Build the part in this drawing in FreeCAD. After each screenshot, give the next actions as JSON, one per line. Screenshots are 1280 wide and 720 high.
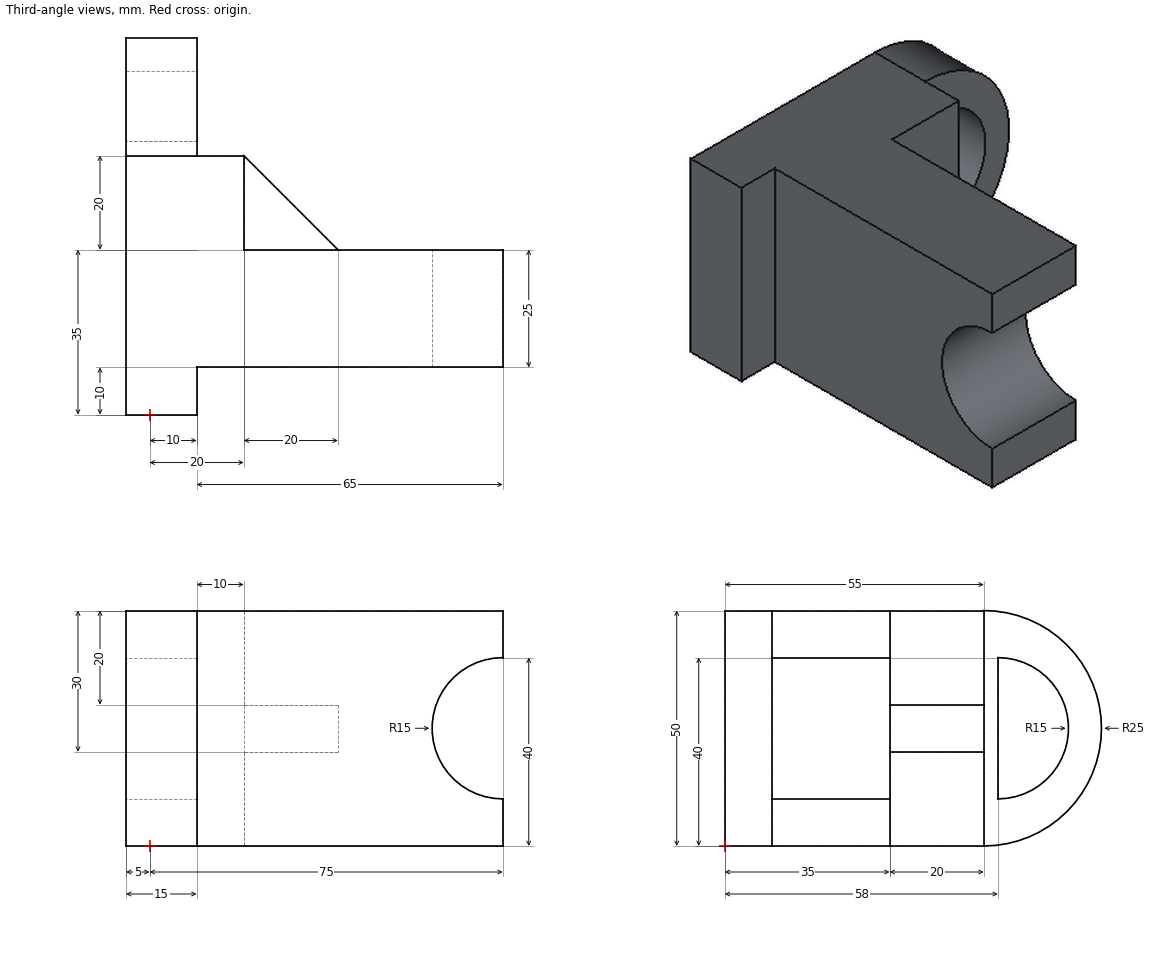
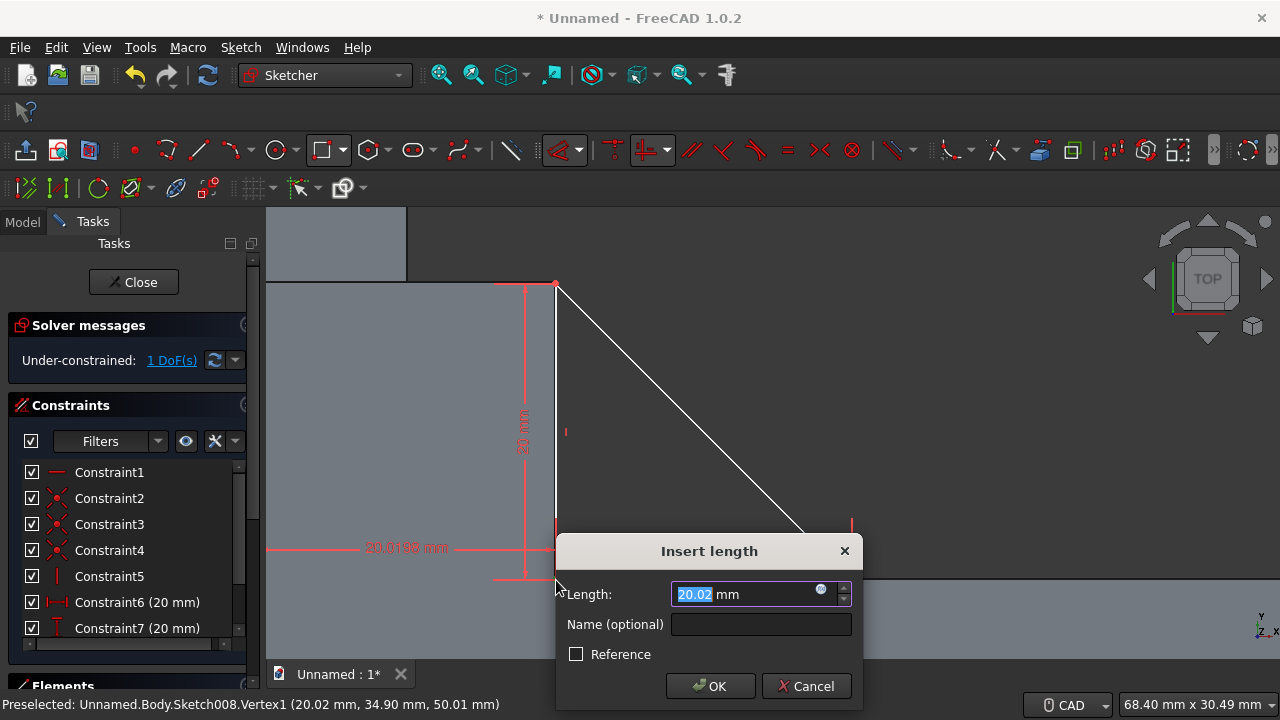
{"action": "type", "text": "20"}
{"action": "key", "text": "Return"}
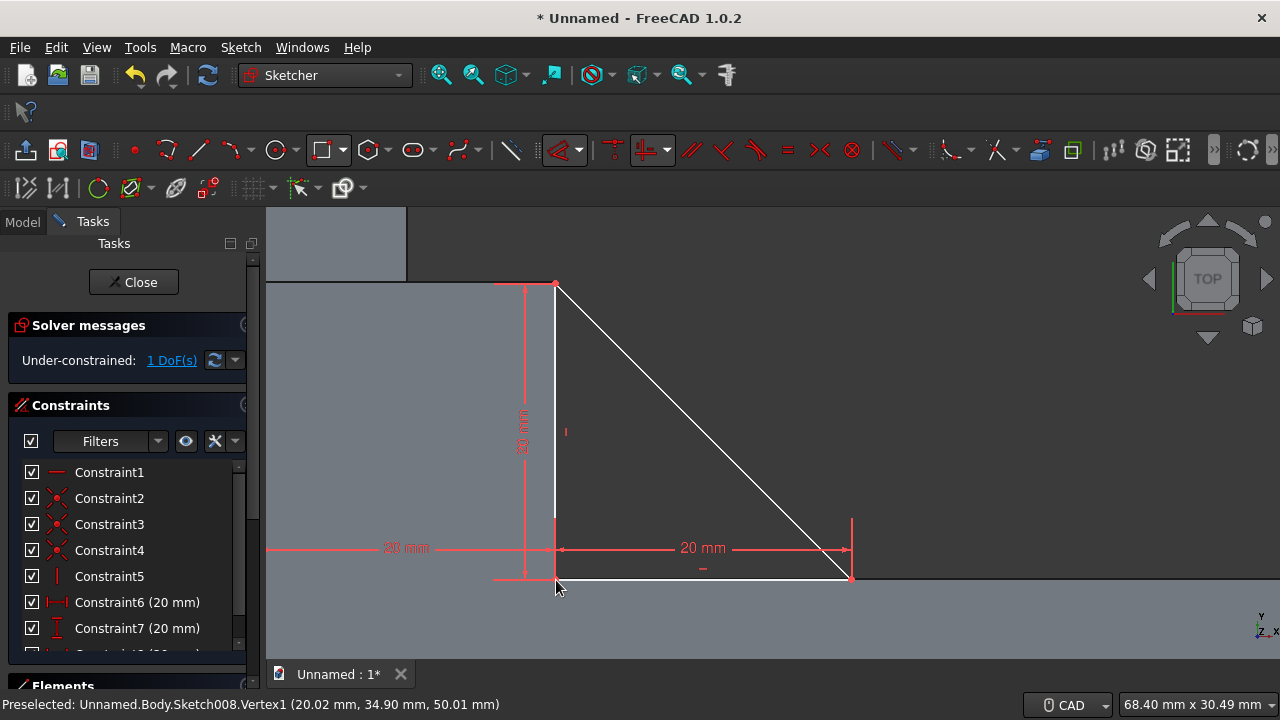
{"action": "left_click", "coordinate": [555, 580]}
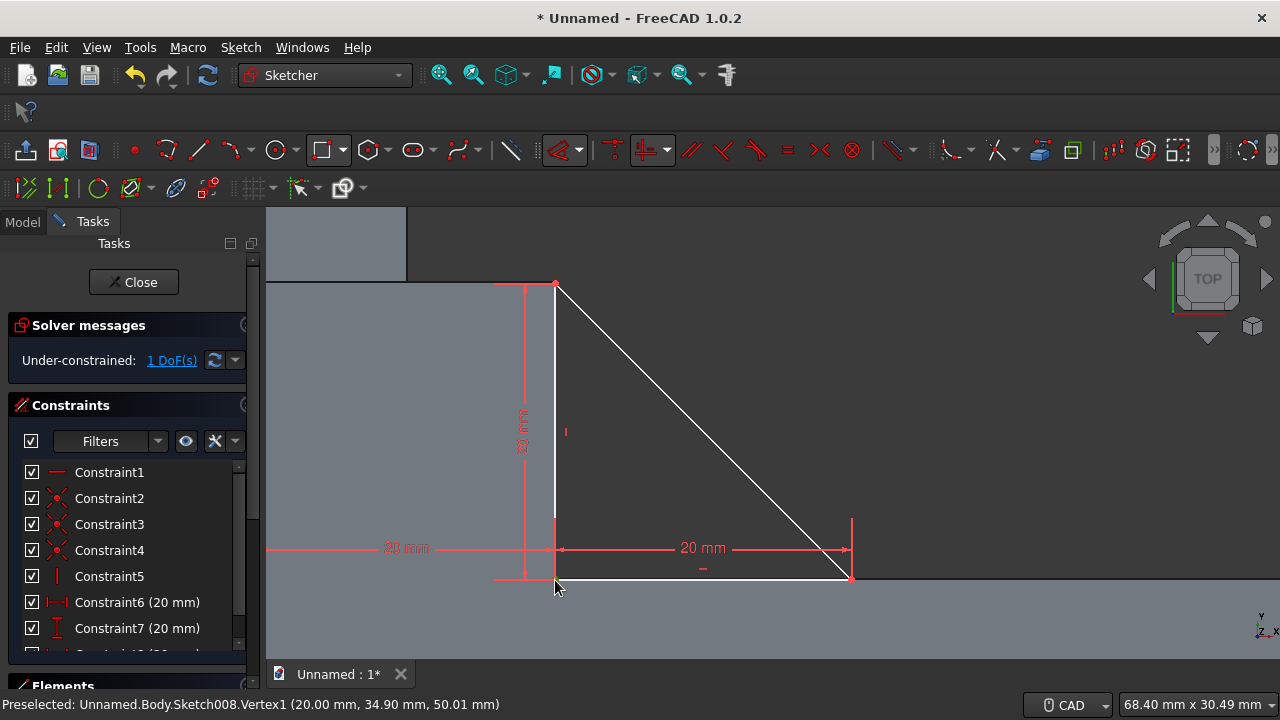
{"action": "key", "text": "i"}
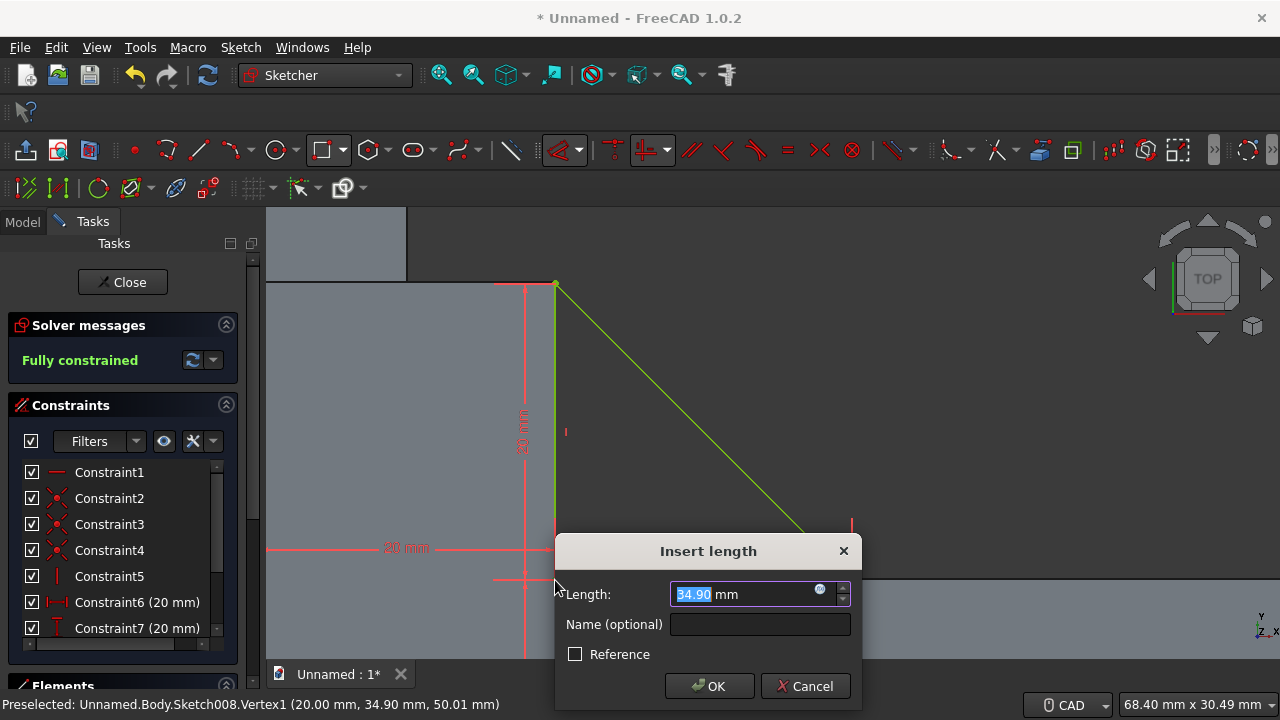
{"action": "type", "text": "35"}
{"action": "key", "text": "Return"}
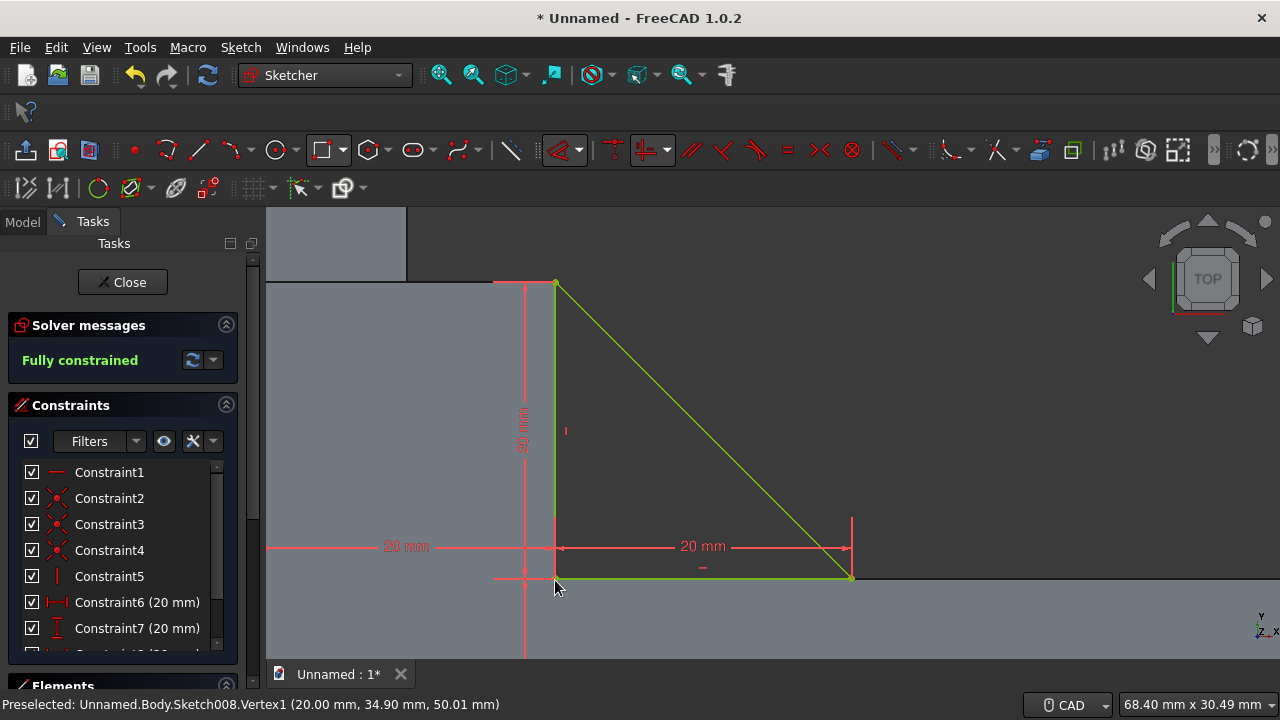
{"action": "left_click", "coordinate": [123, 282]}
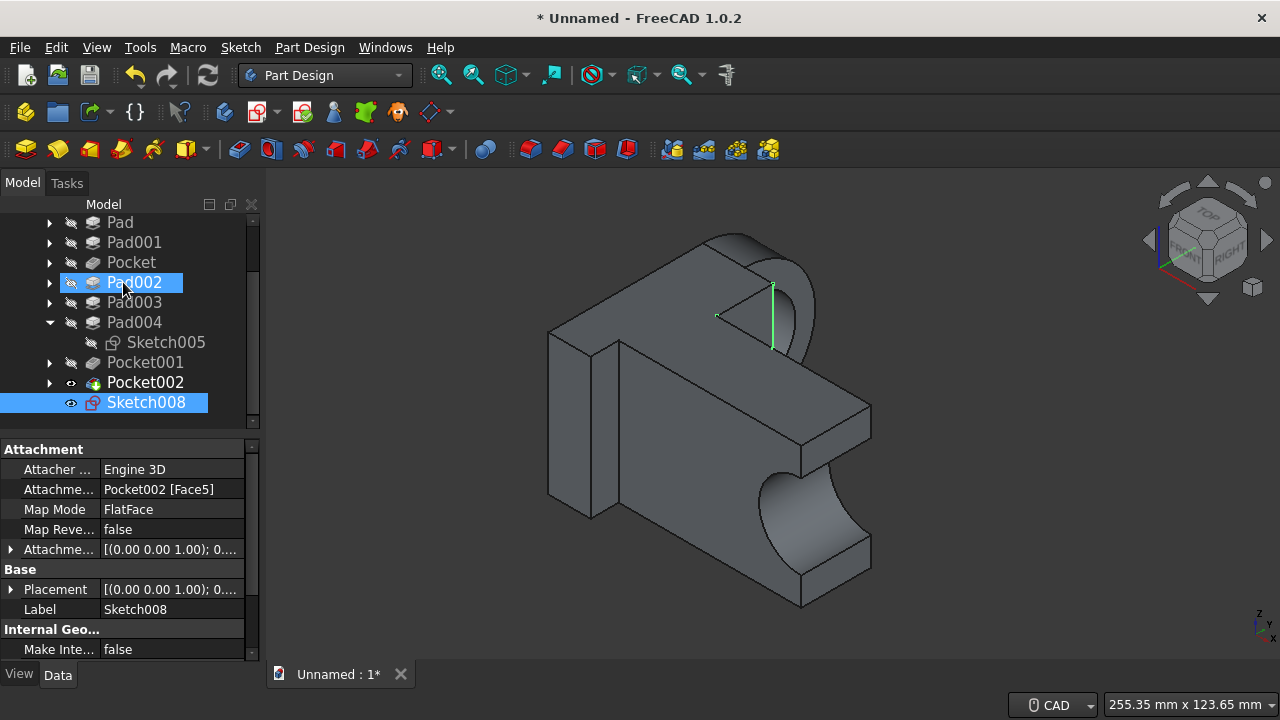
{"action": "left_click", "coordinate": [26, 150]}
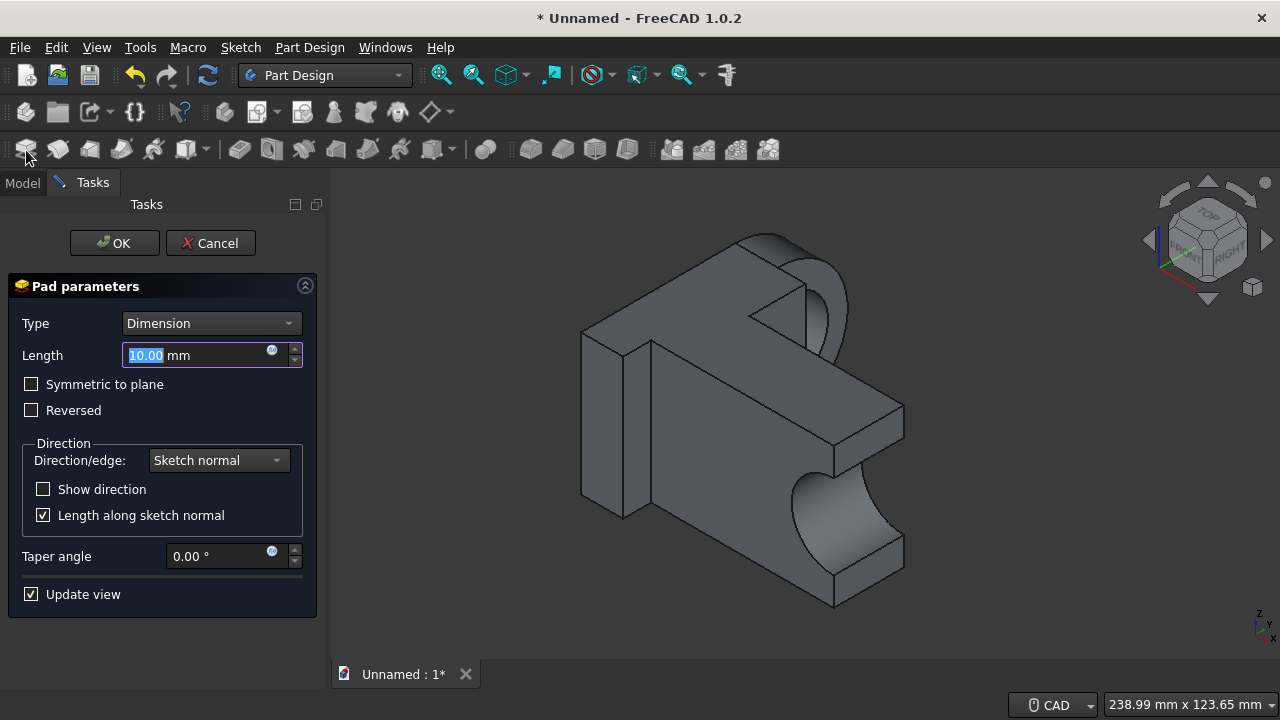
{"action": "type", "text": "30"}
{"action": "key", "text": "Tab"}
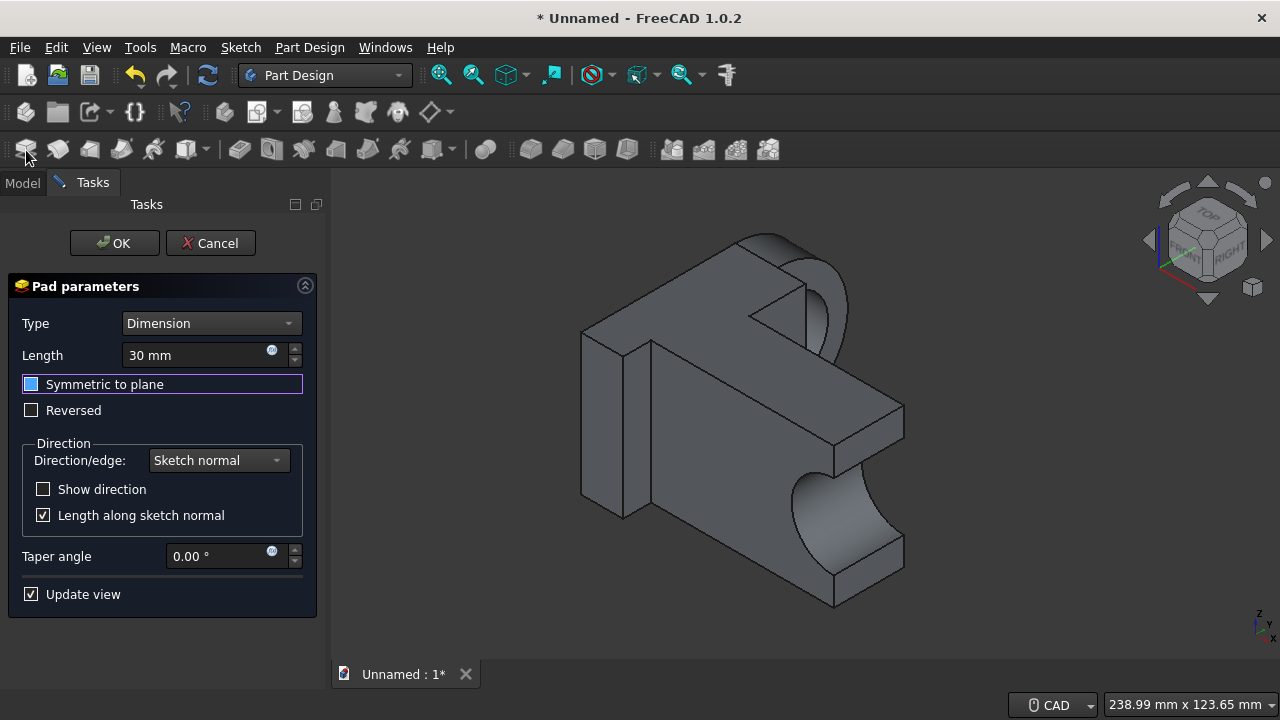
{"action": "left_click", "coordinate": [30, 410]}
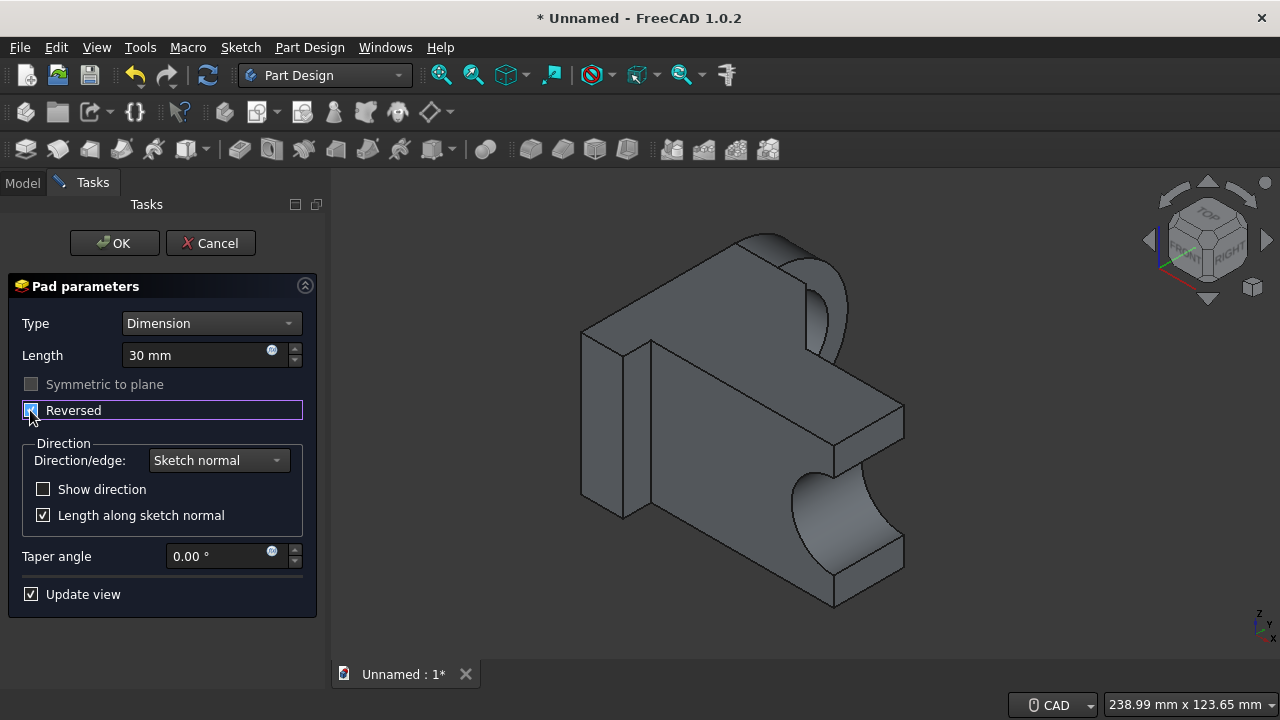
{"action": "left_click", "coordinate": [115, 243]}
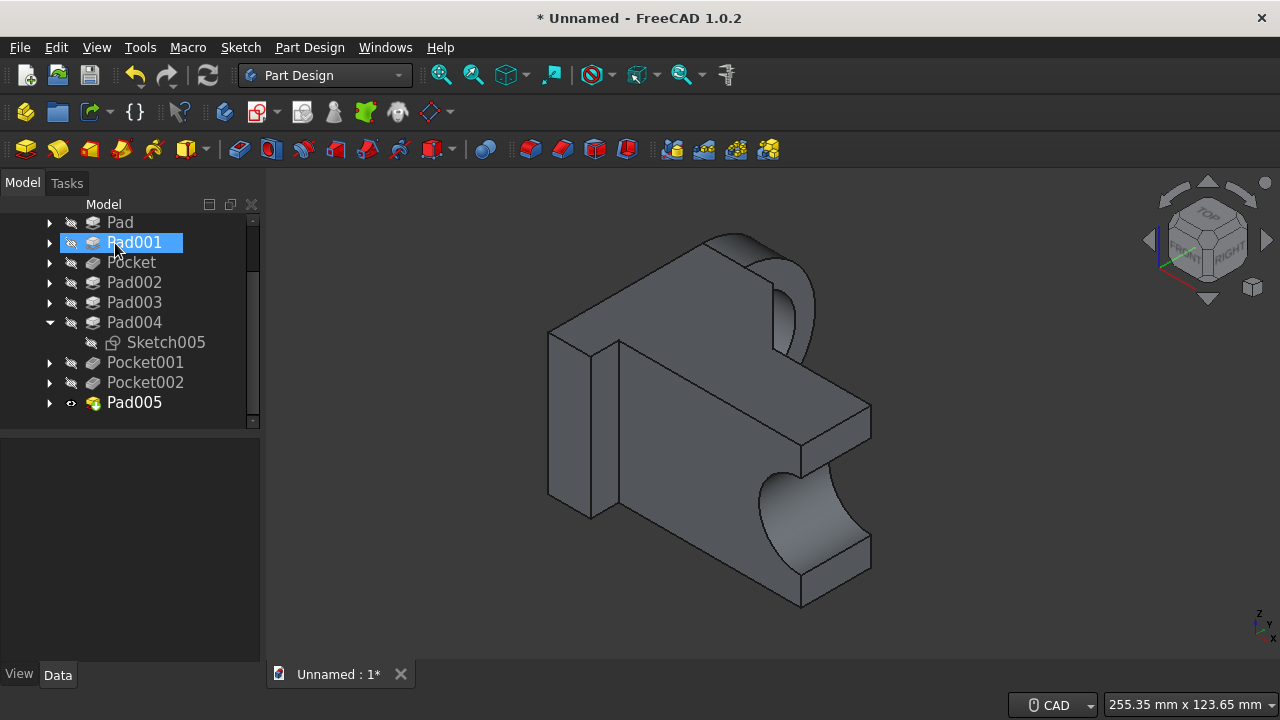
{"action": "left_click", "coordinate": [696, 302]}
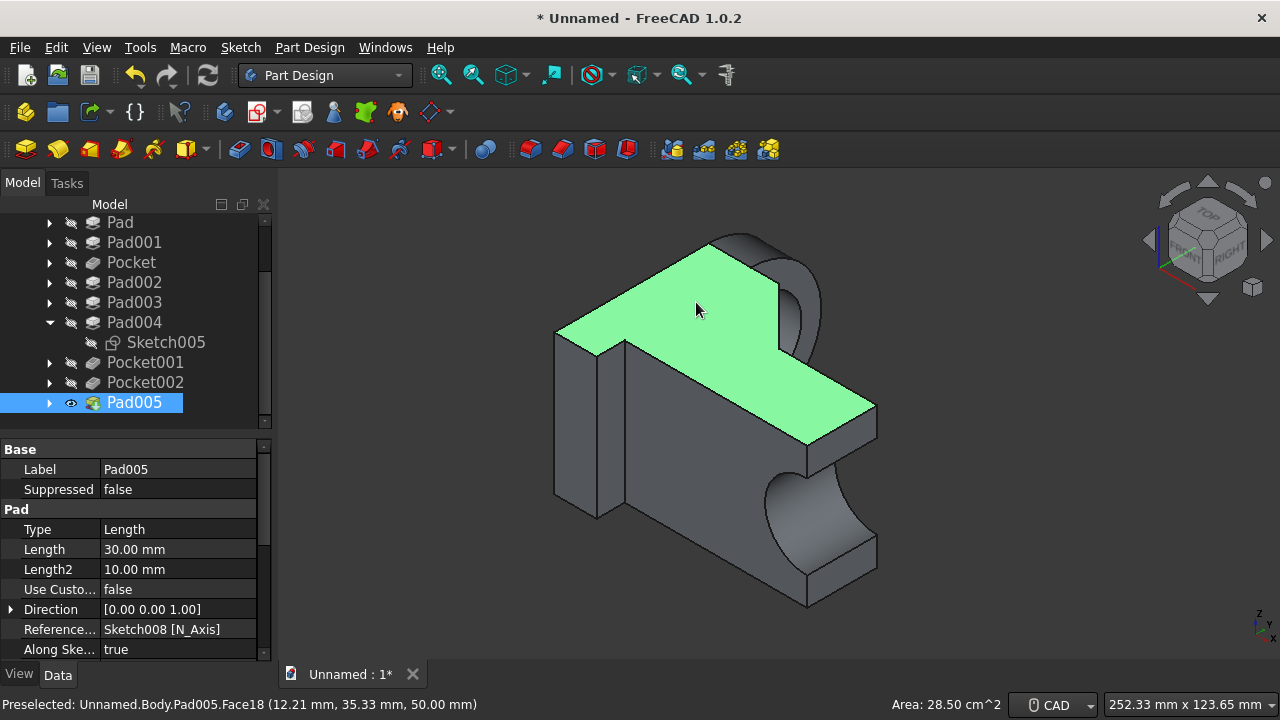
{"action": "left_click", "coordinate": [258, 112]}